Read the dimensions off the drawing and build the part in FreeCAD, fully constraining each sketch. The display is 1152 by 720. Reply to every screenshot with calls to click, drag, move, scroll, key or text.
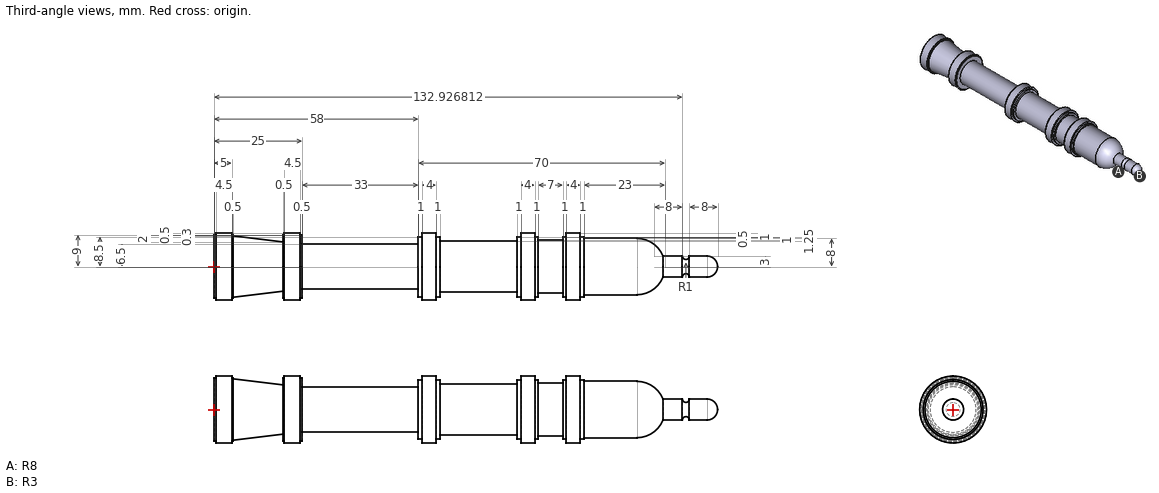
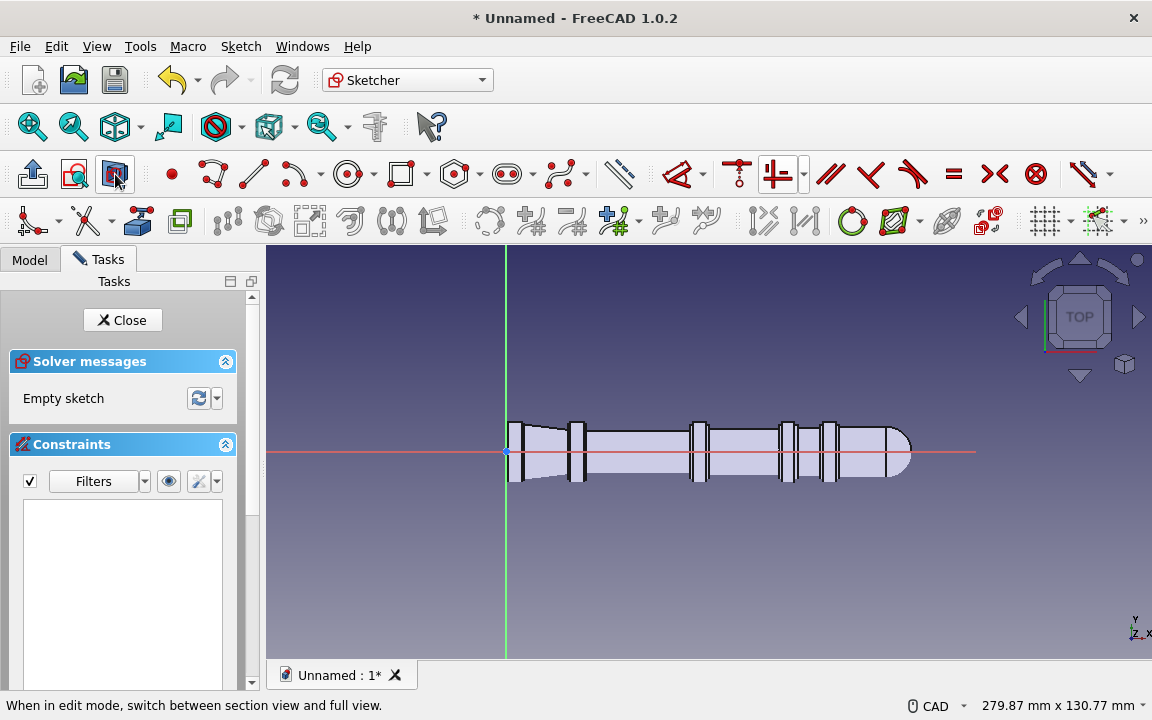
scroll(966, 447, up, 11)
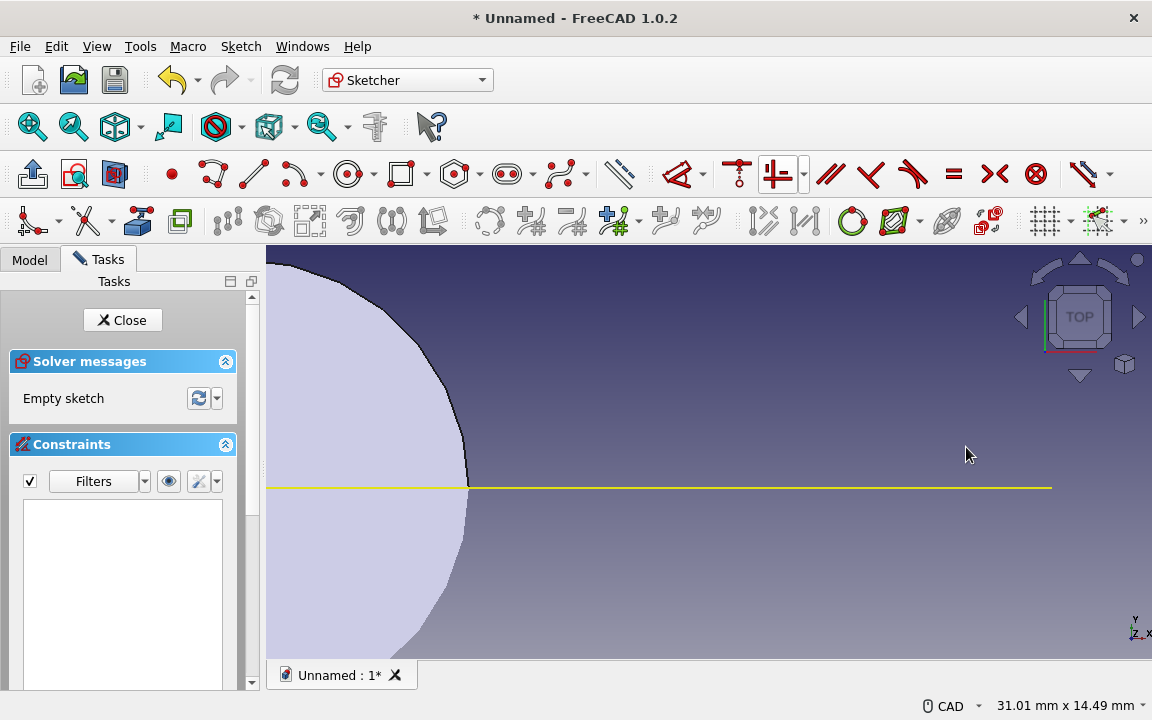
click(213, 174)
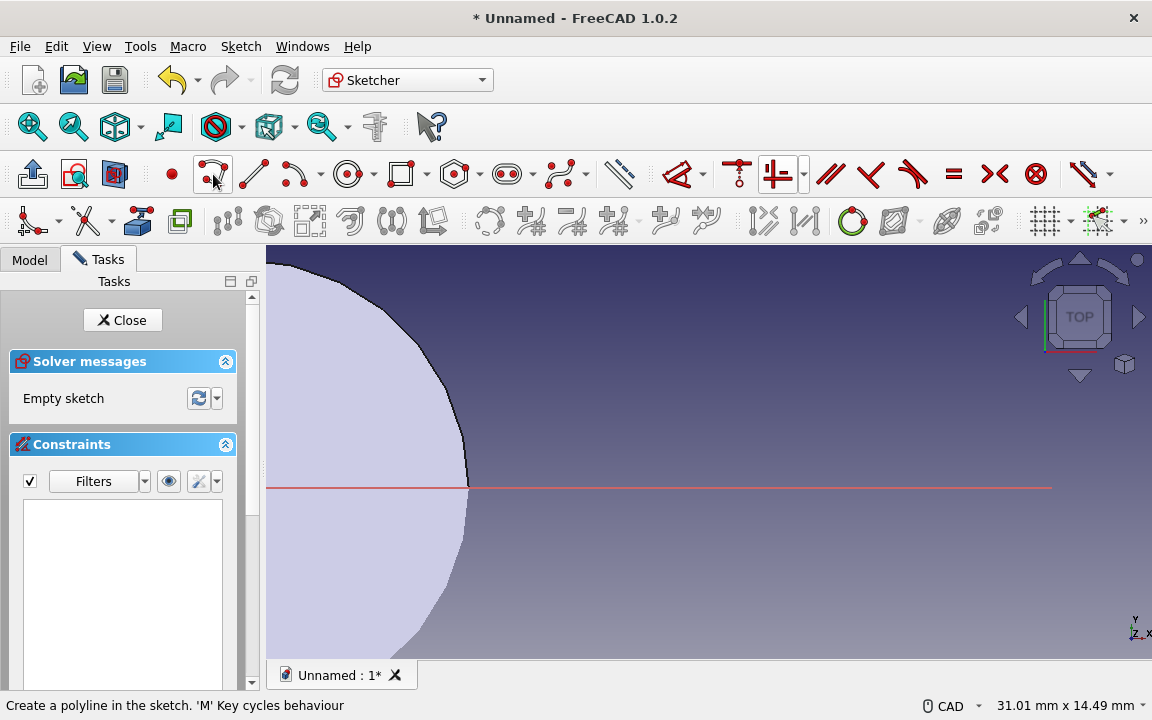
click(610, 402)
click(381, 402)
click(381, 488)
click(895, 479)
click(895, 402)
click(667, 402)
right_click(667, 402)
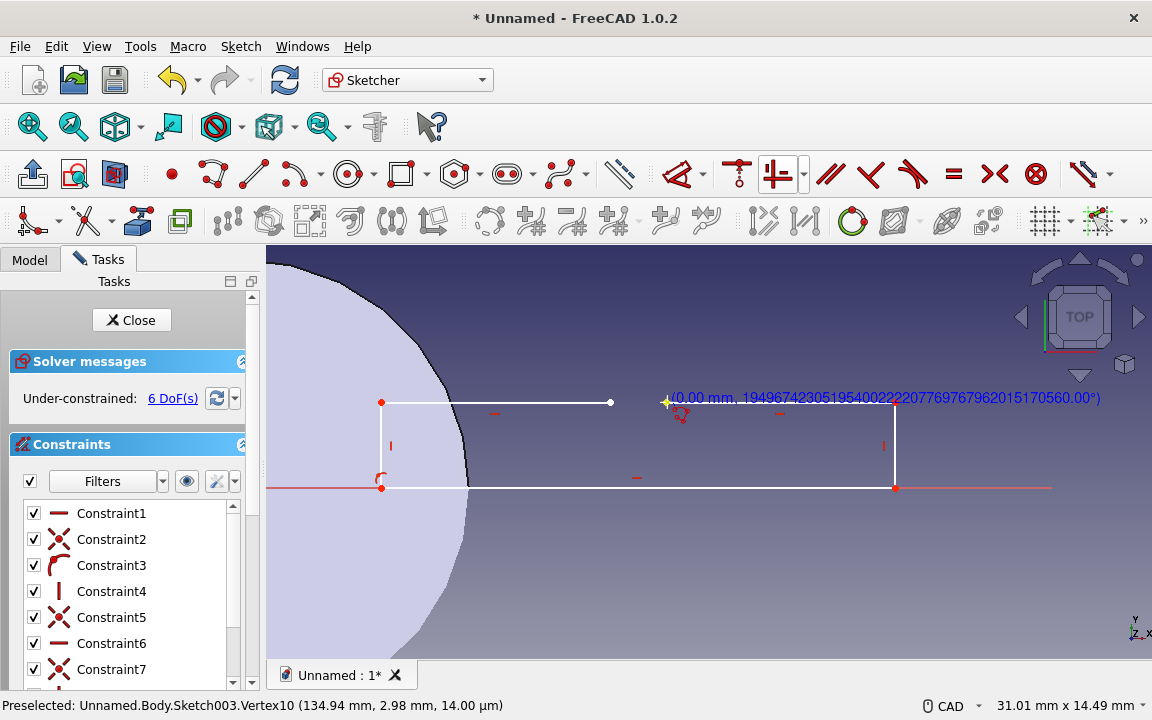
key(g)
key(3)
key(a)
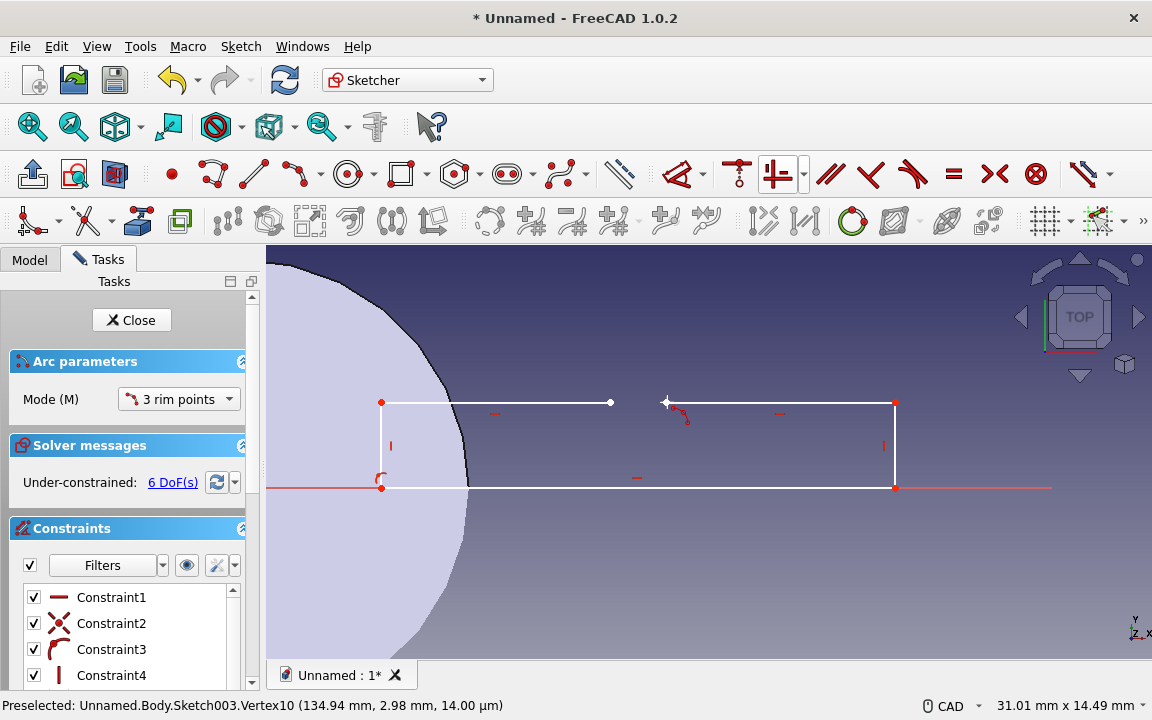
click(667, 403)
click(610, 403)
click(638, 431)
key(Escape)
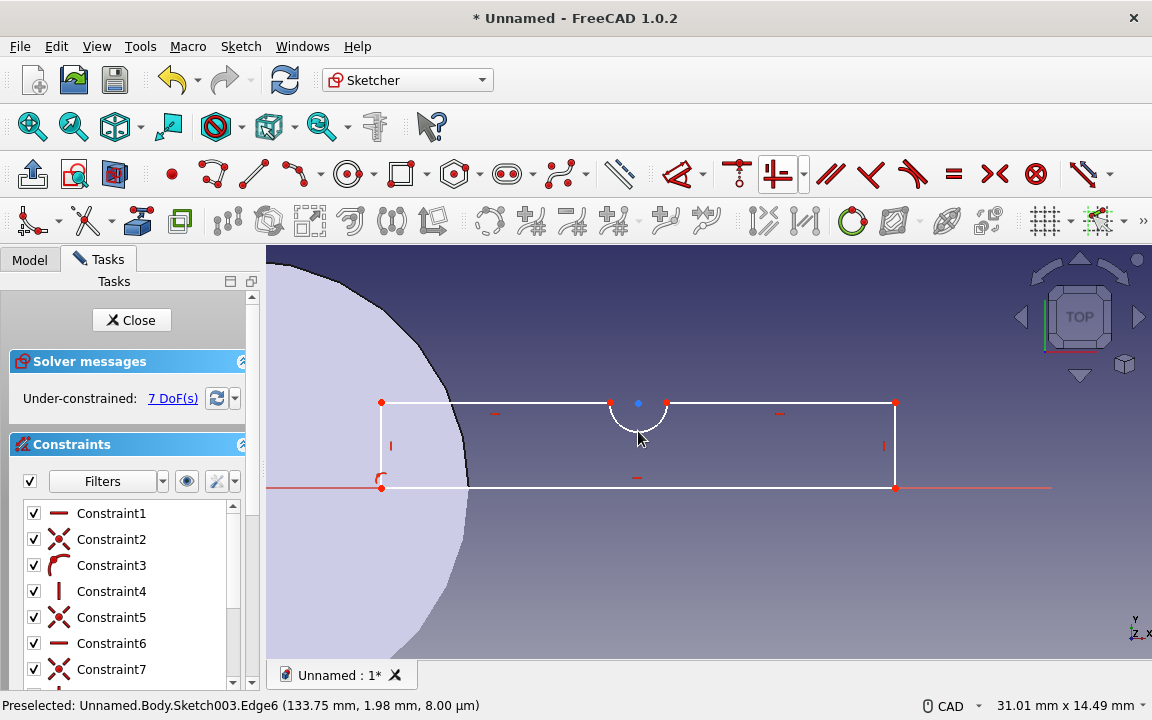
click(676, 174)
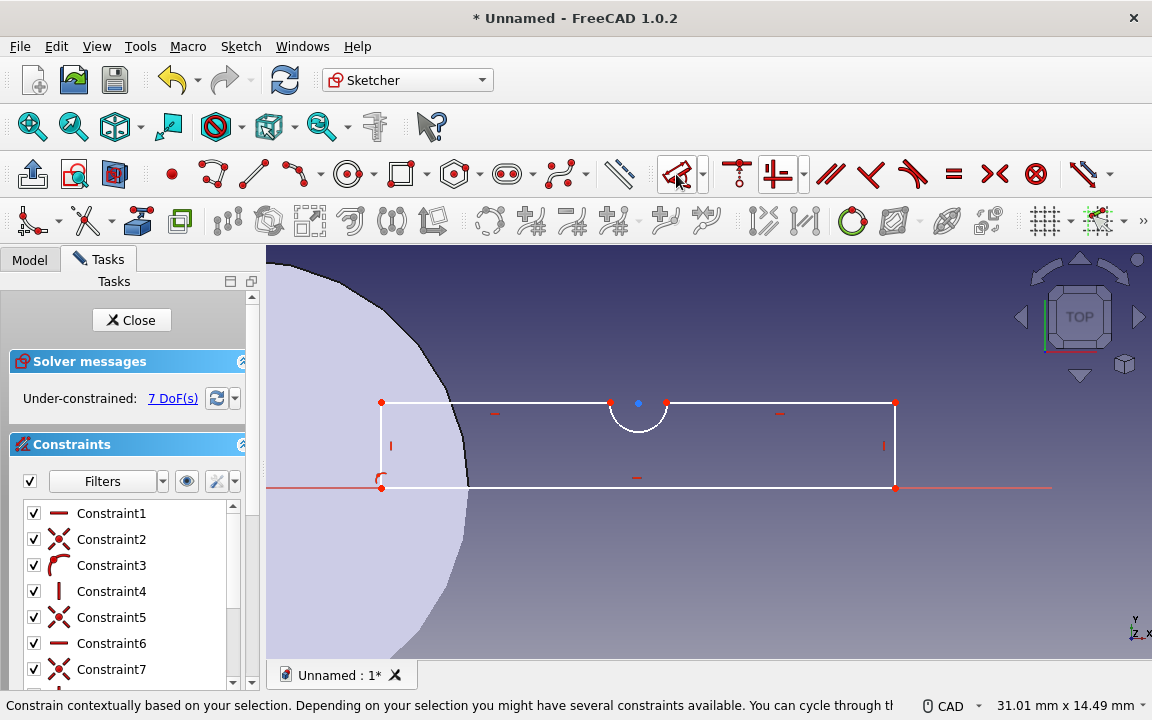
scroll(622, 426, up, 2)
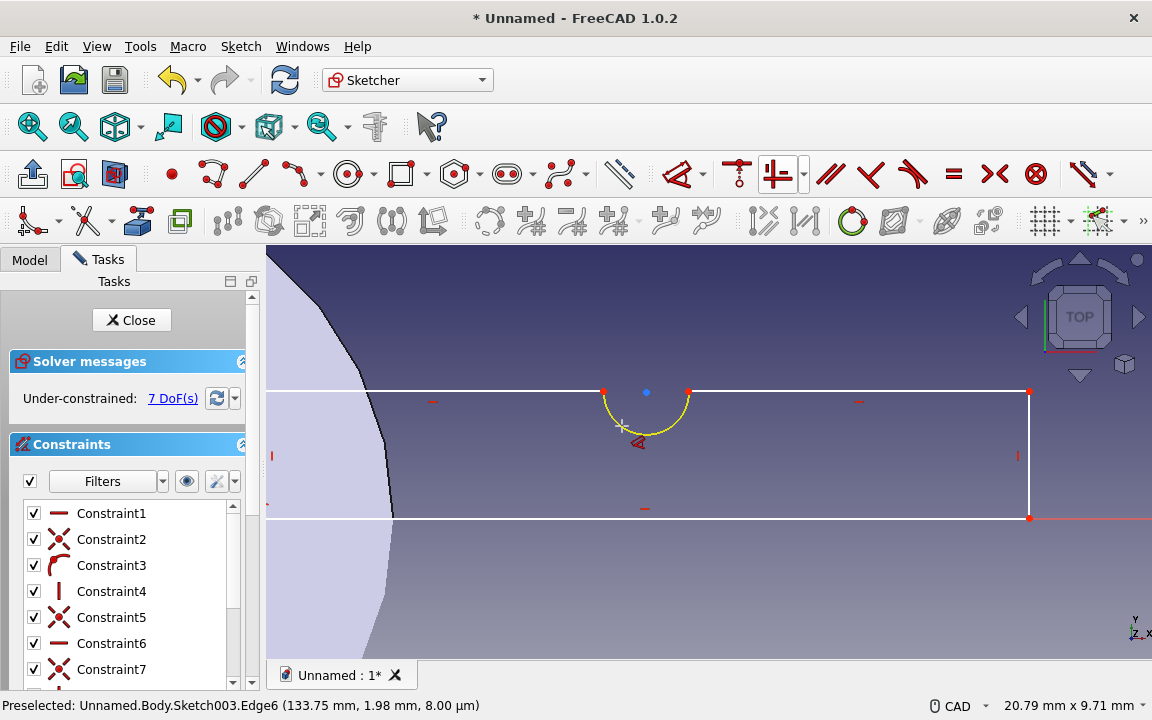
click(621, 426)
click(602, 452)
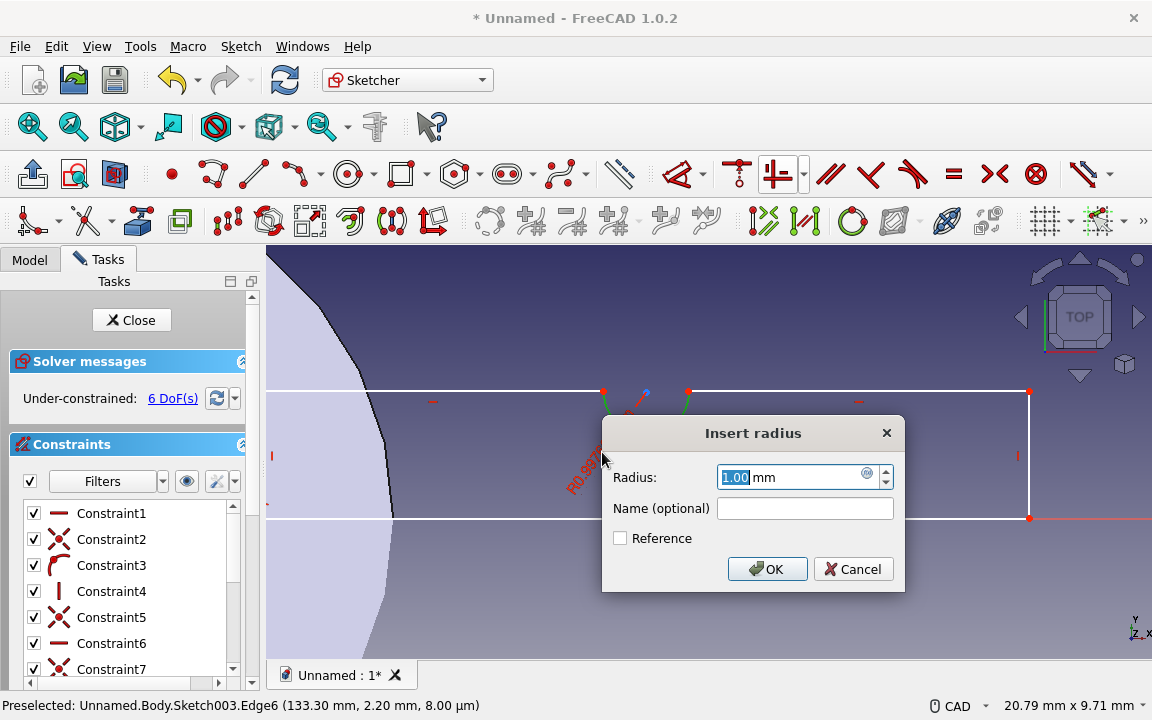
text(1)
key(Return)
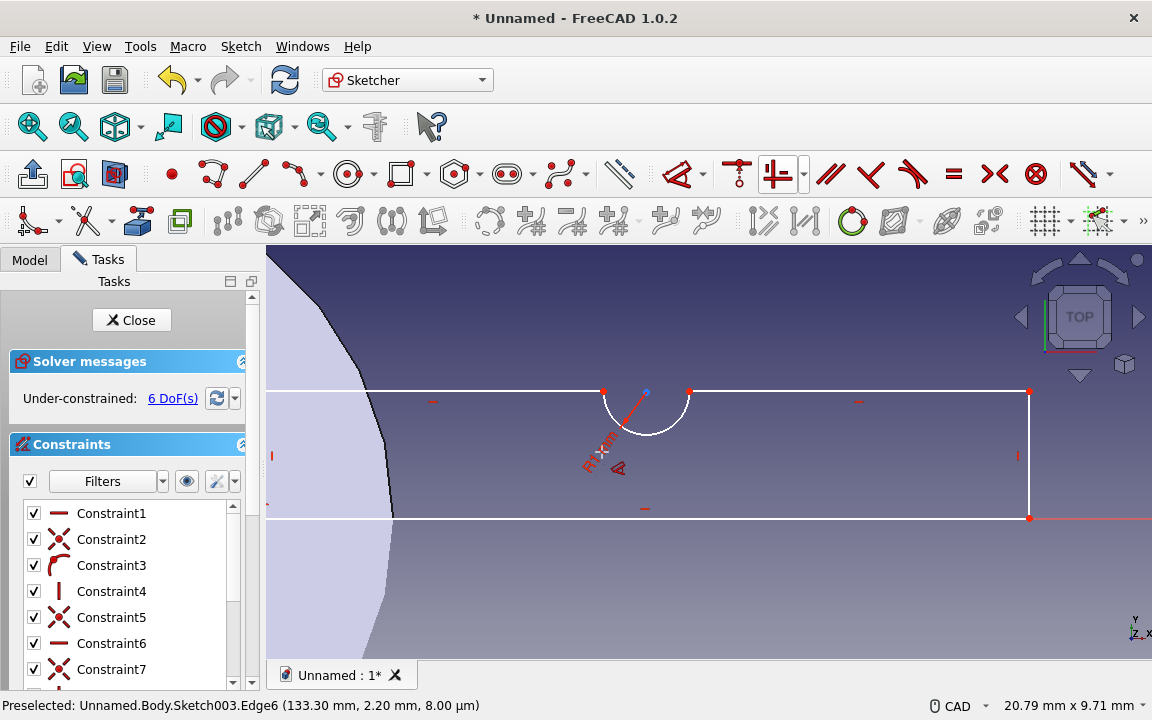
click(501, 391)
click(449, 357)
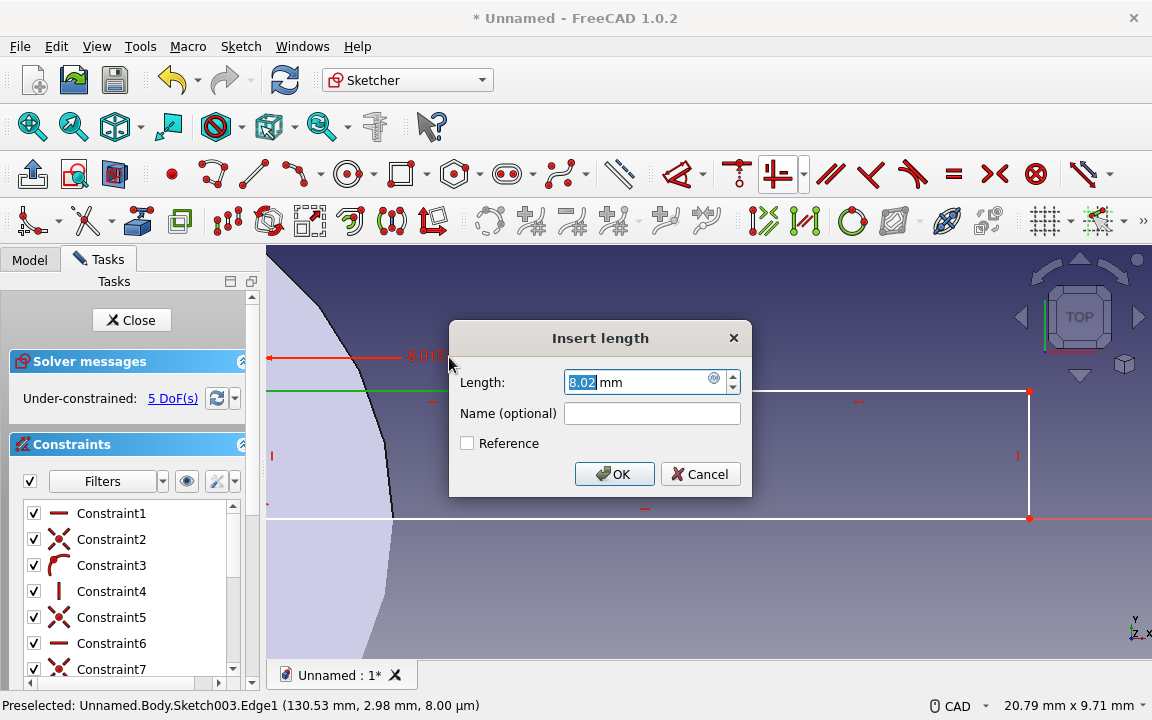
text(8)
key(Return)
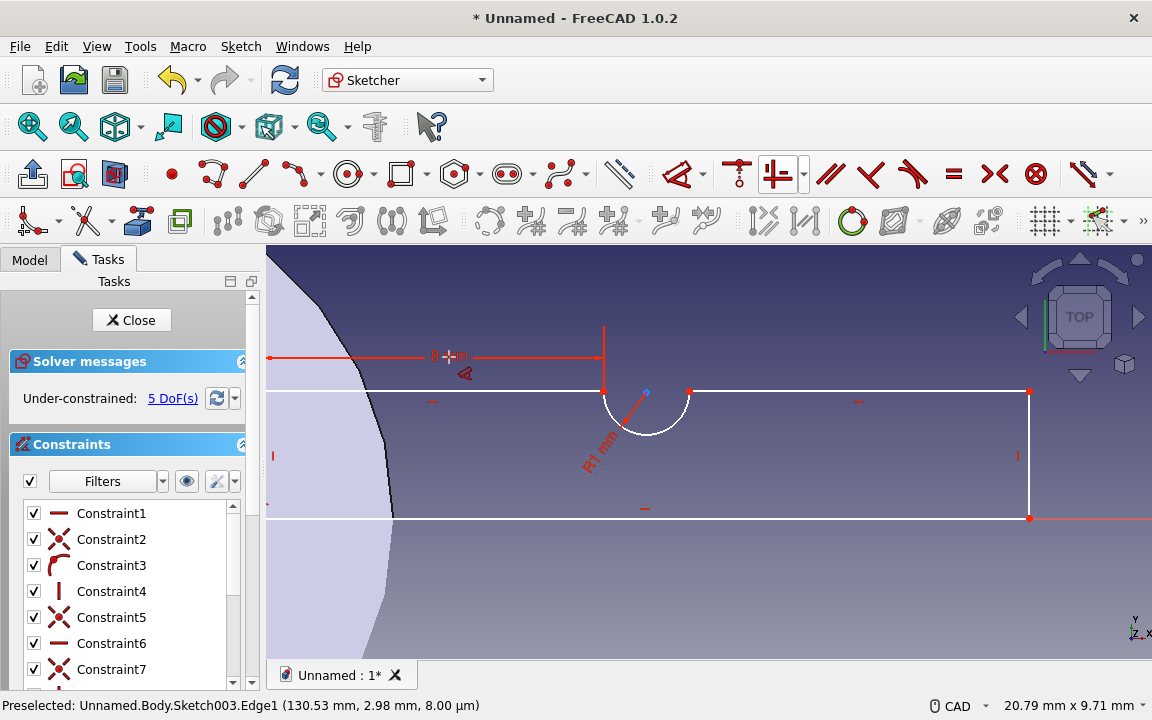
scroll(630, 447, down, 2)